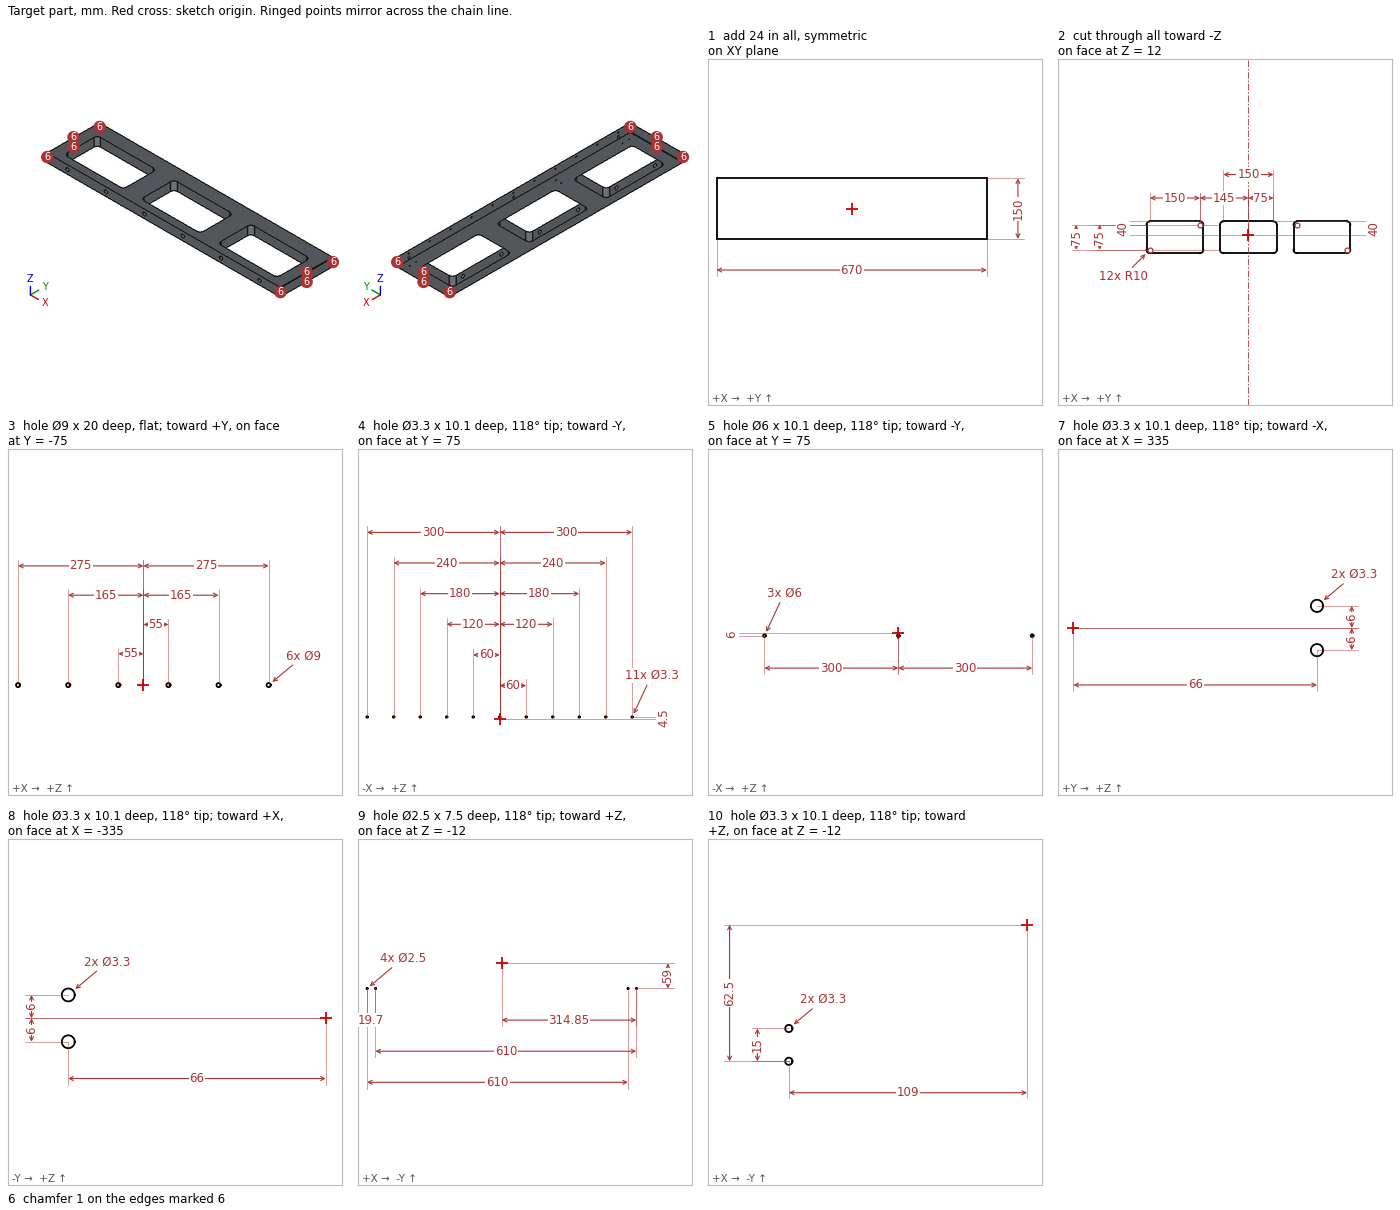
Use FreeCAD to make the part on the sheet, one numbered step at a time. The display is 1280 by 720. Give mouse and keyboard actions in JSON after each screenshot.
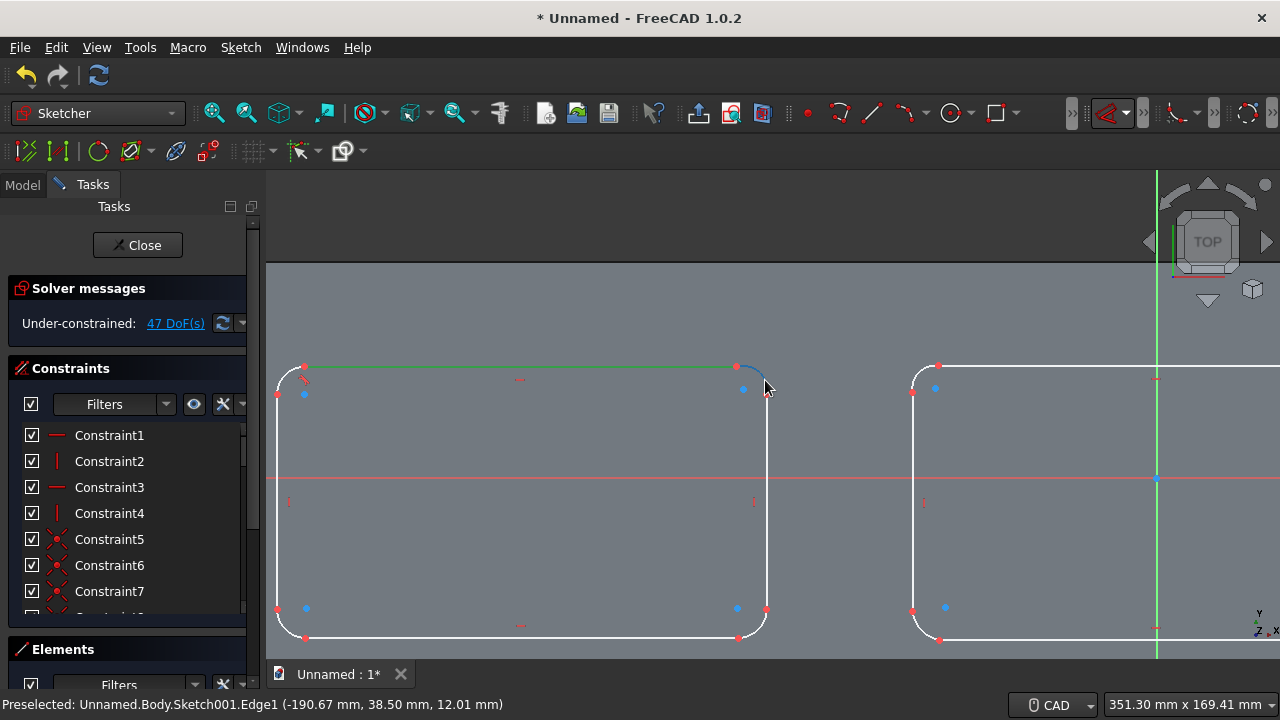
{"action": "left_click", "coordinate": [765, 380]}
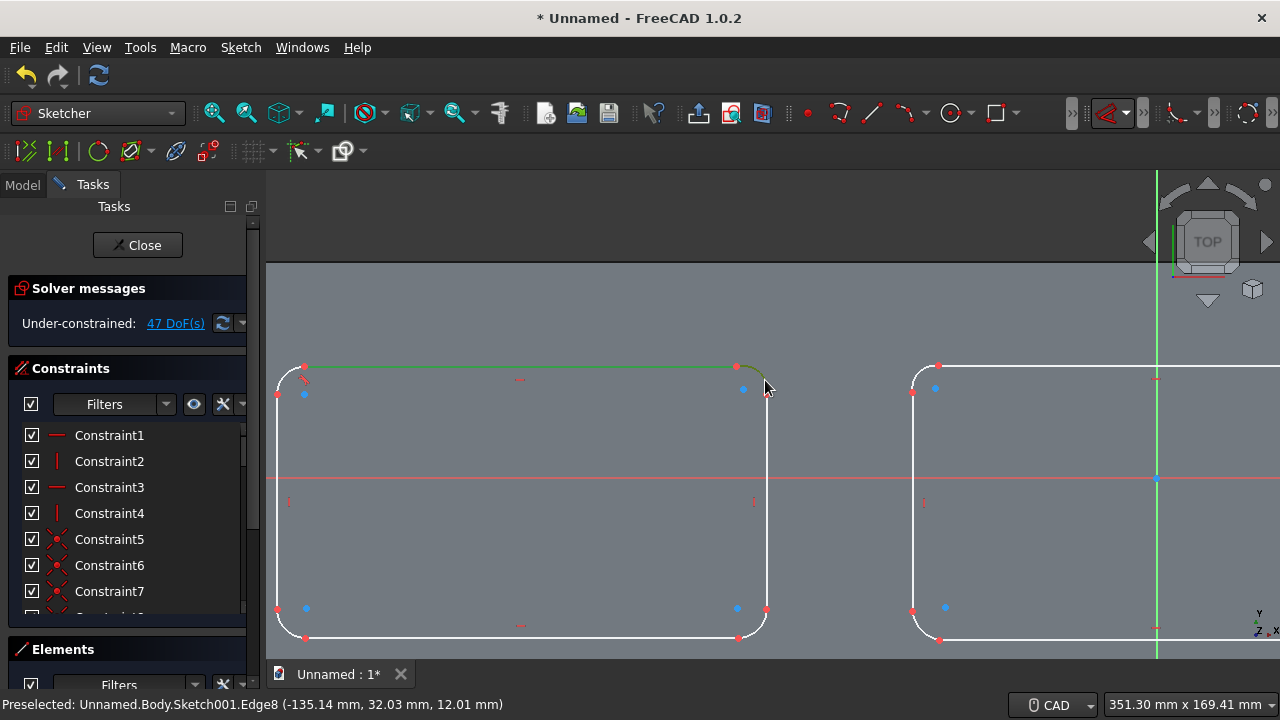
{"action": "key", "text": "t"}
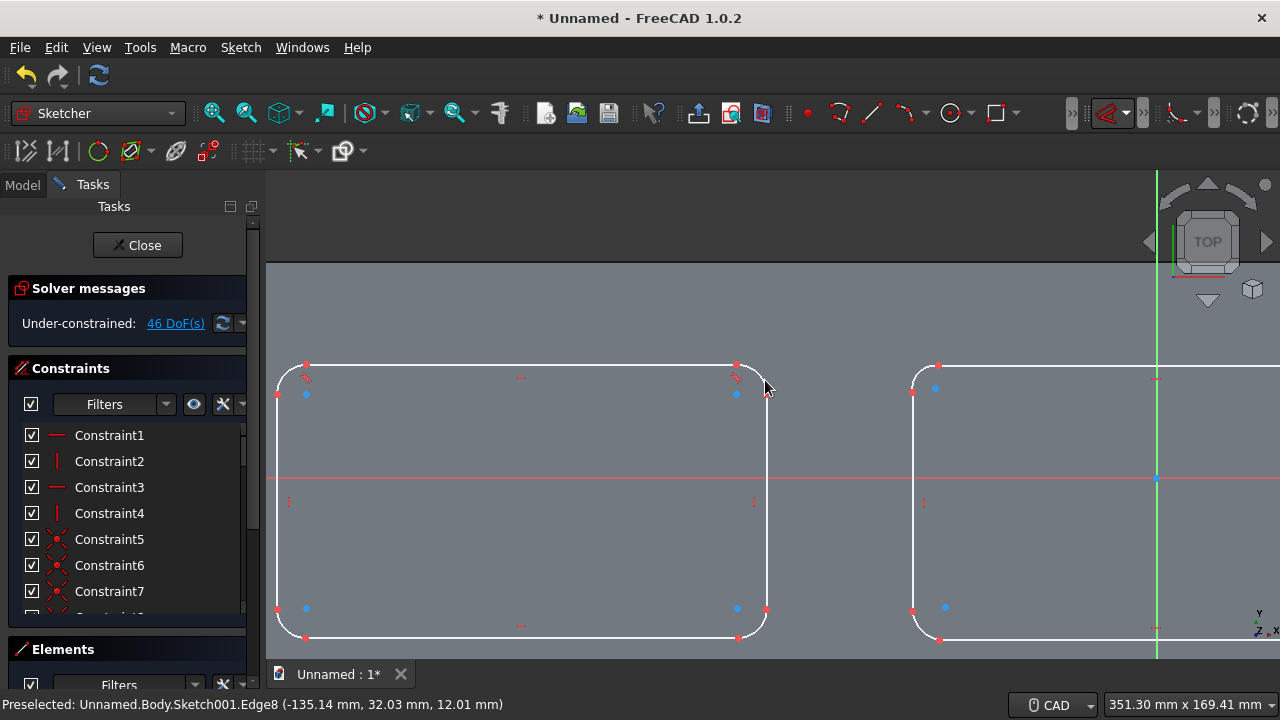
{"action": "scroll", "coordinate": [509, 378], "scroll_direction": "down", "scroll_amount": 6}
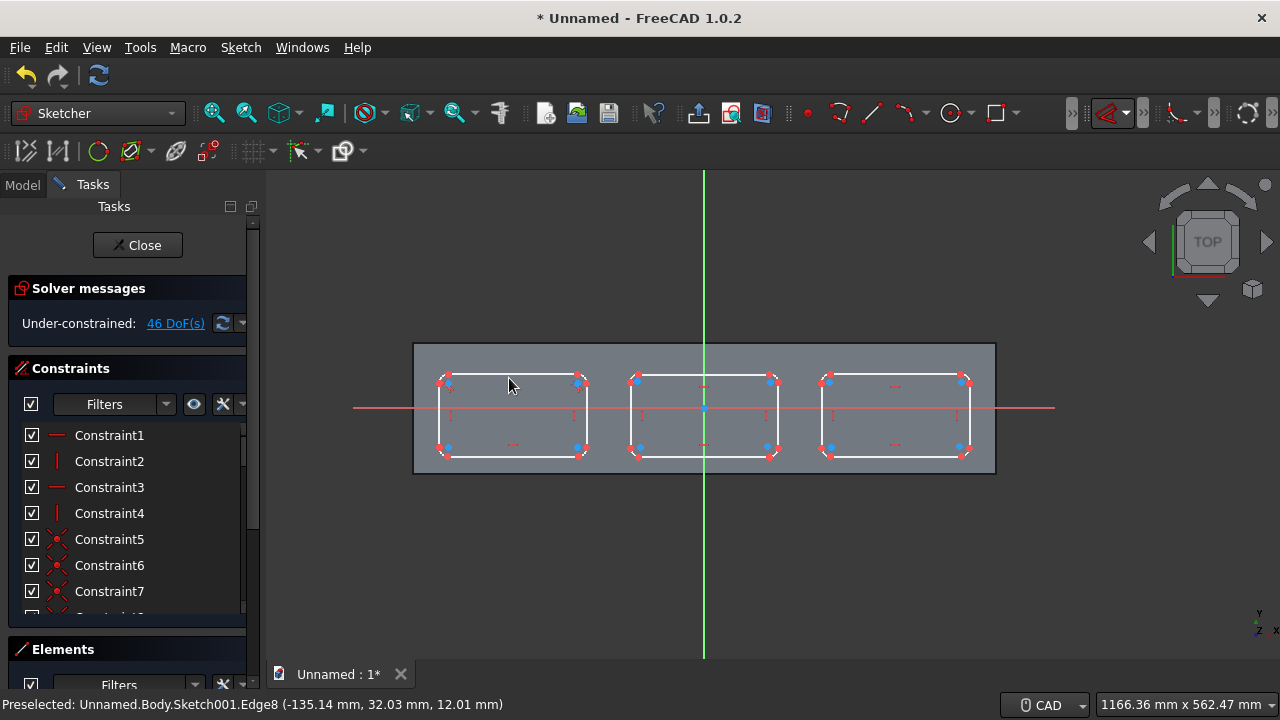
{"action": "scroll", "coordinate": [439, 403], "scroll_direction": "up", "scroll_amount": 5}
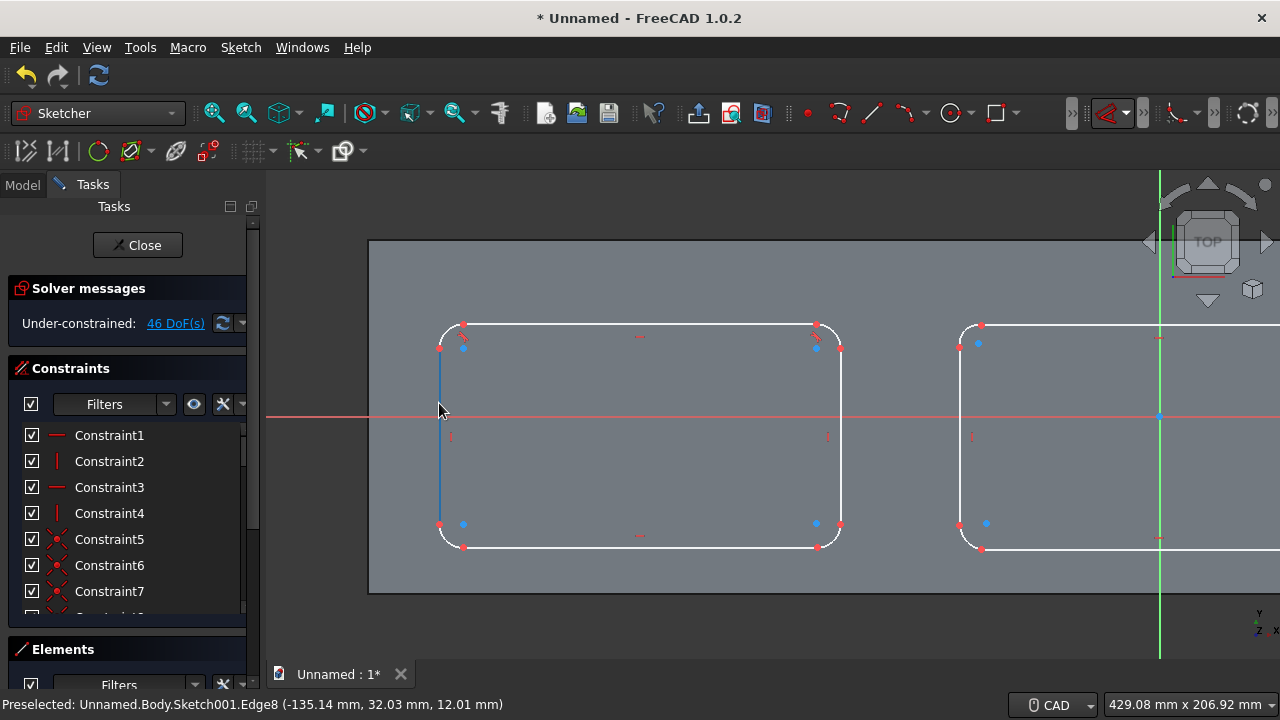
{"action": "left_click", "coordinate": [440, 401]}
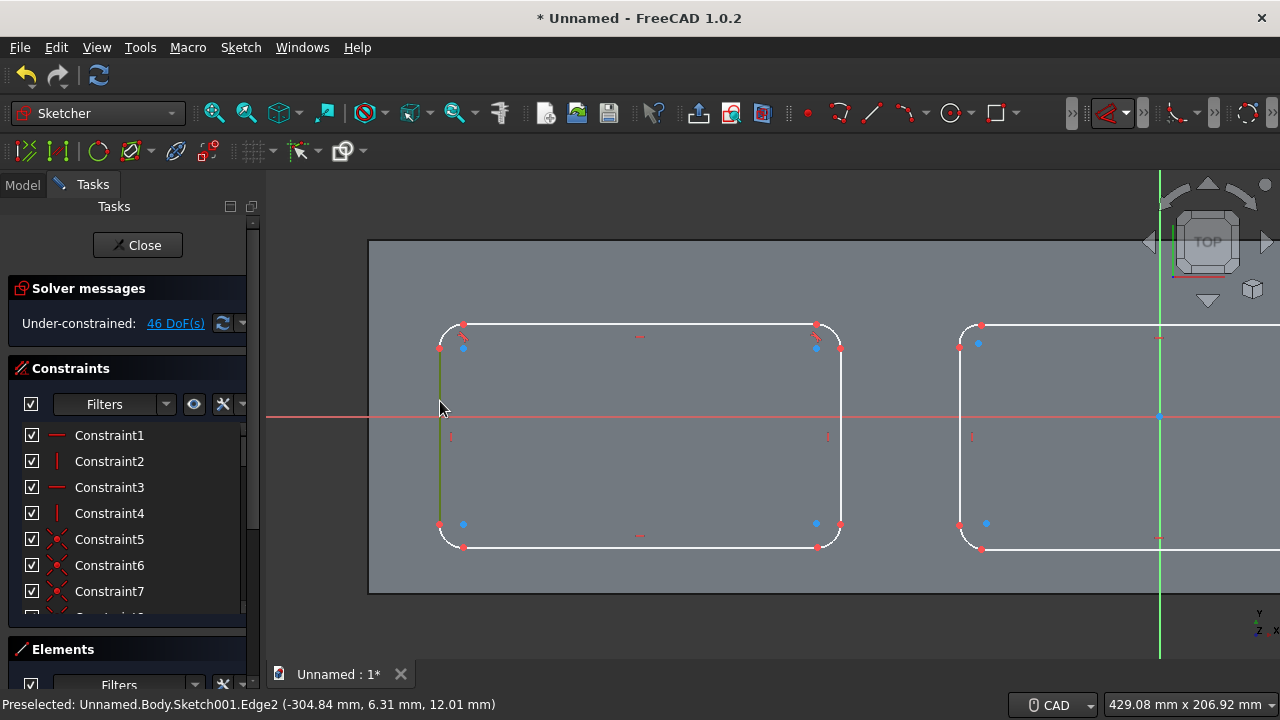
{"action": "scroll", "coordinate": [453, 327], "scroll_direction": "up", "scroll_amount": 2}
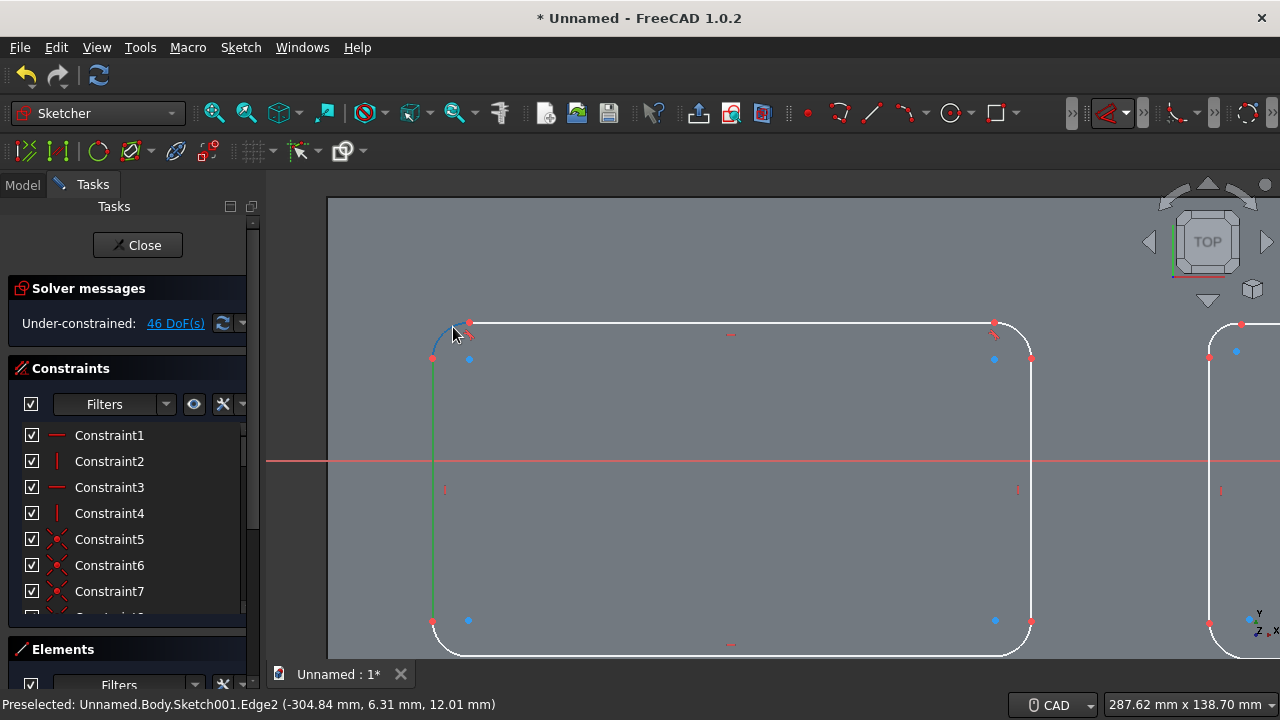
{"action": "left_click", "coordinate": [453, 327]}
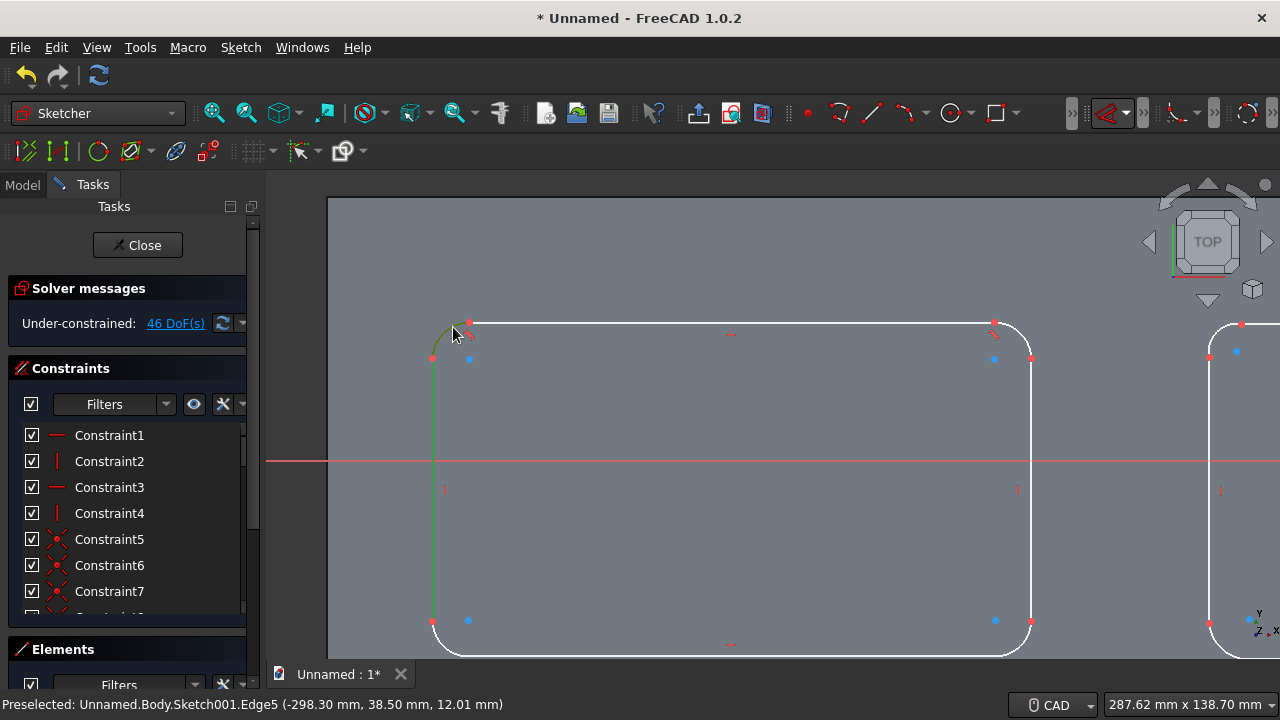
{"action": "key", "text": "t"}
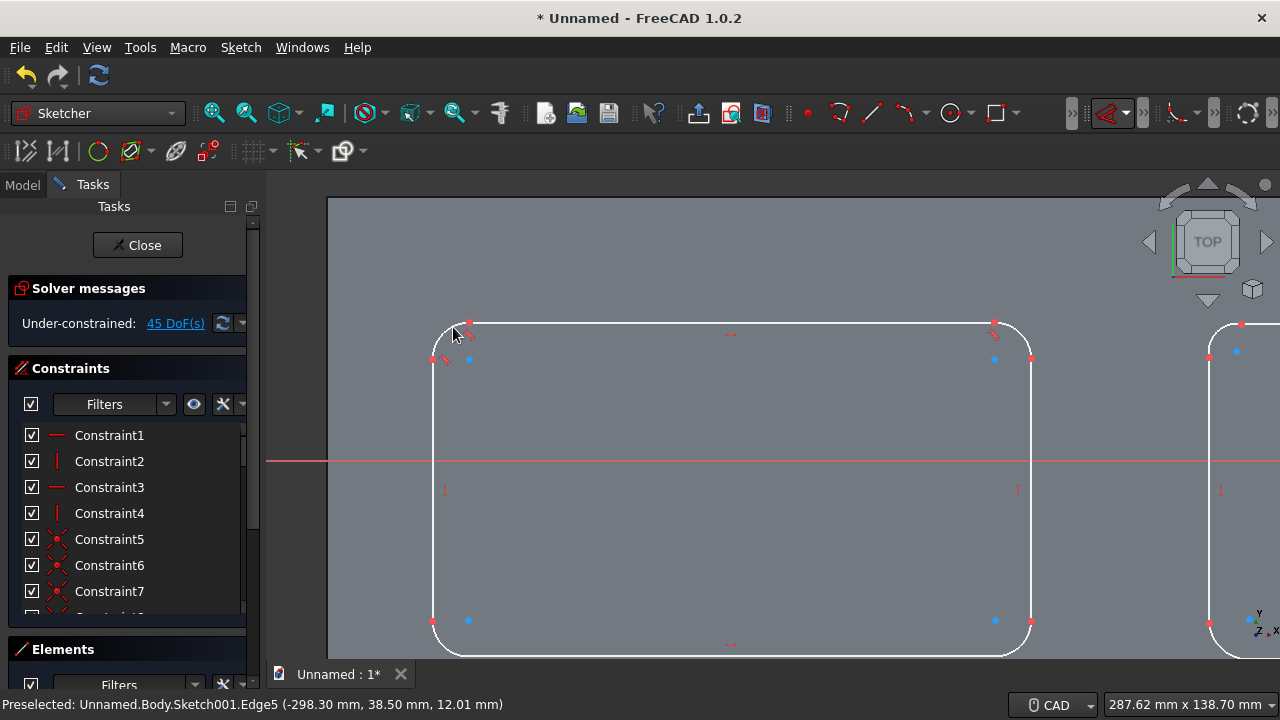
{"action": "left_click", "coordinate": [433, 438]}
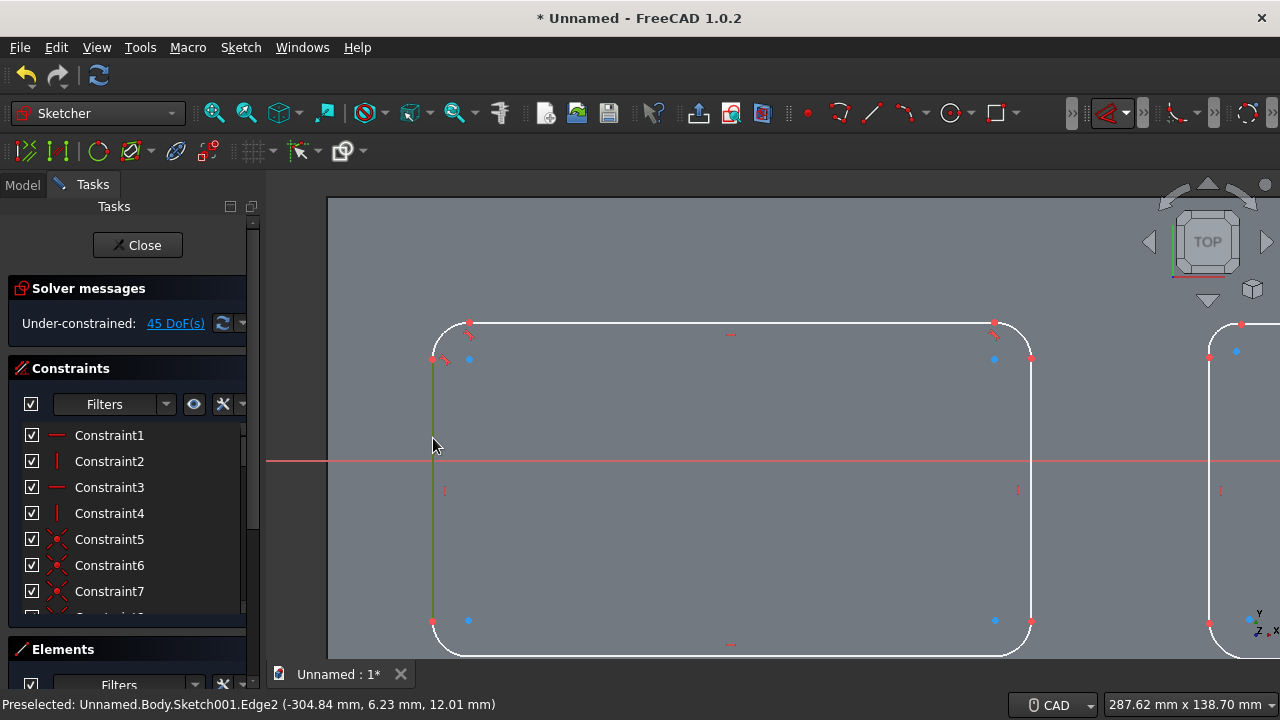
{"action": "scroll", "coordinate": [442, 391], "scroll_direction": "down", "scroll_amount": 7}